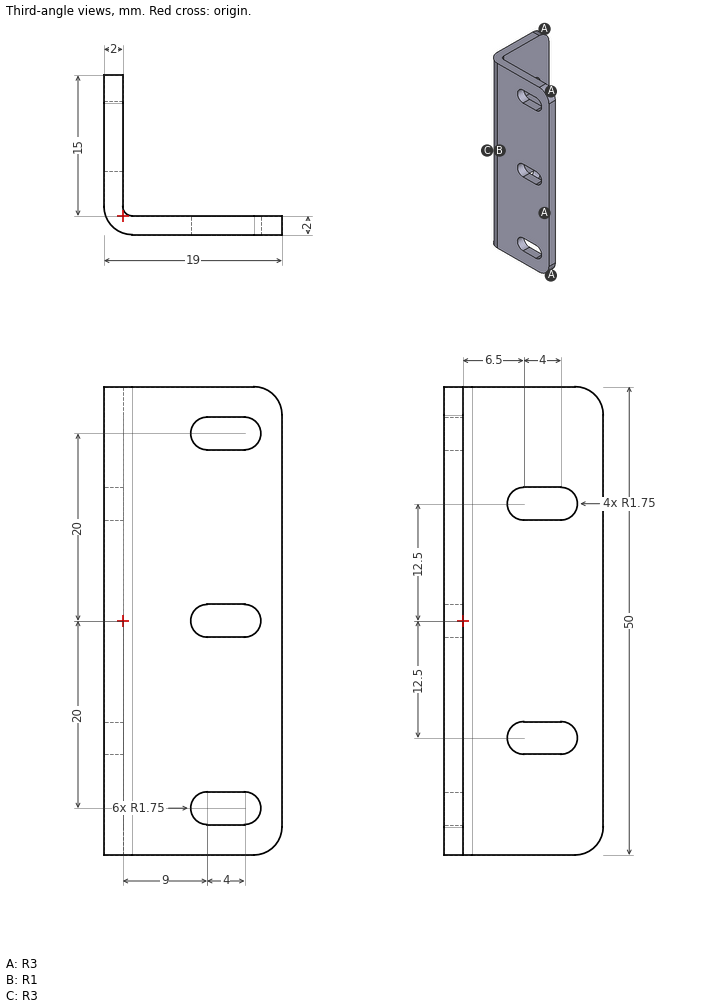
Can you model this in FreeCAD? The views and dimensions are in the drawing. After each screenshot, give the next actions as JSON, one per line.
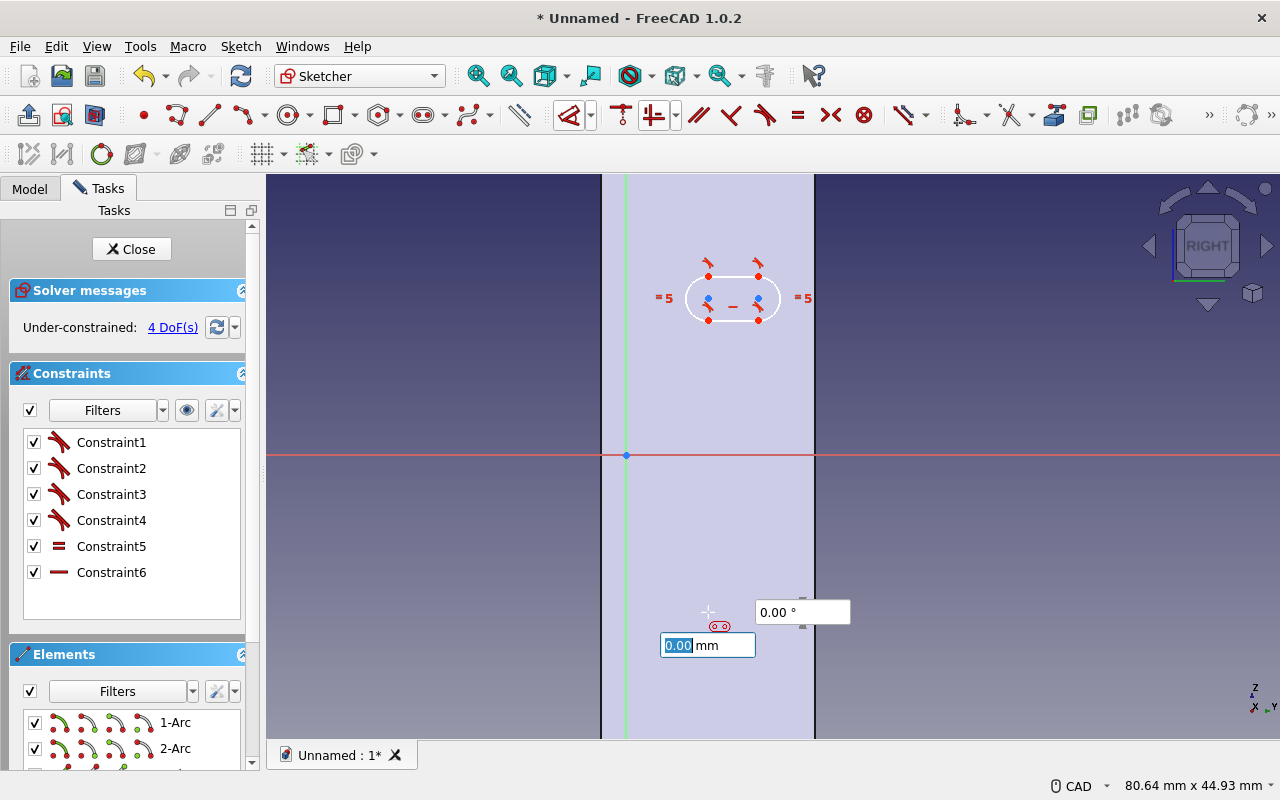
{"action": "left_click", "coordinate": [758, 612]}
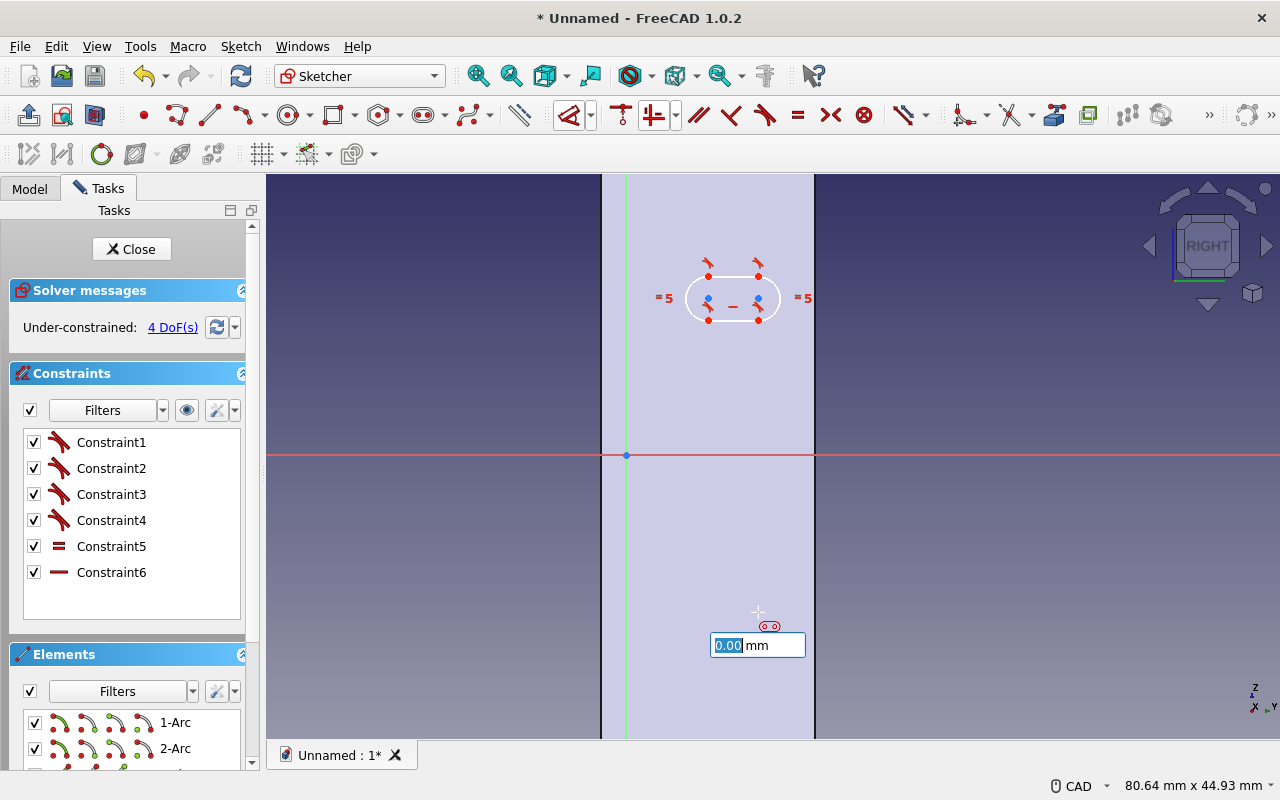
{"action": "left_click", "coordinate": [733, 590]}
{"action": "key", "text": "Escape"}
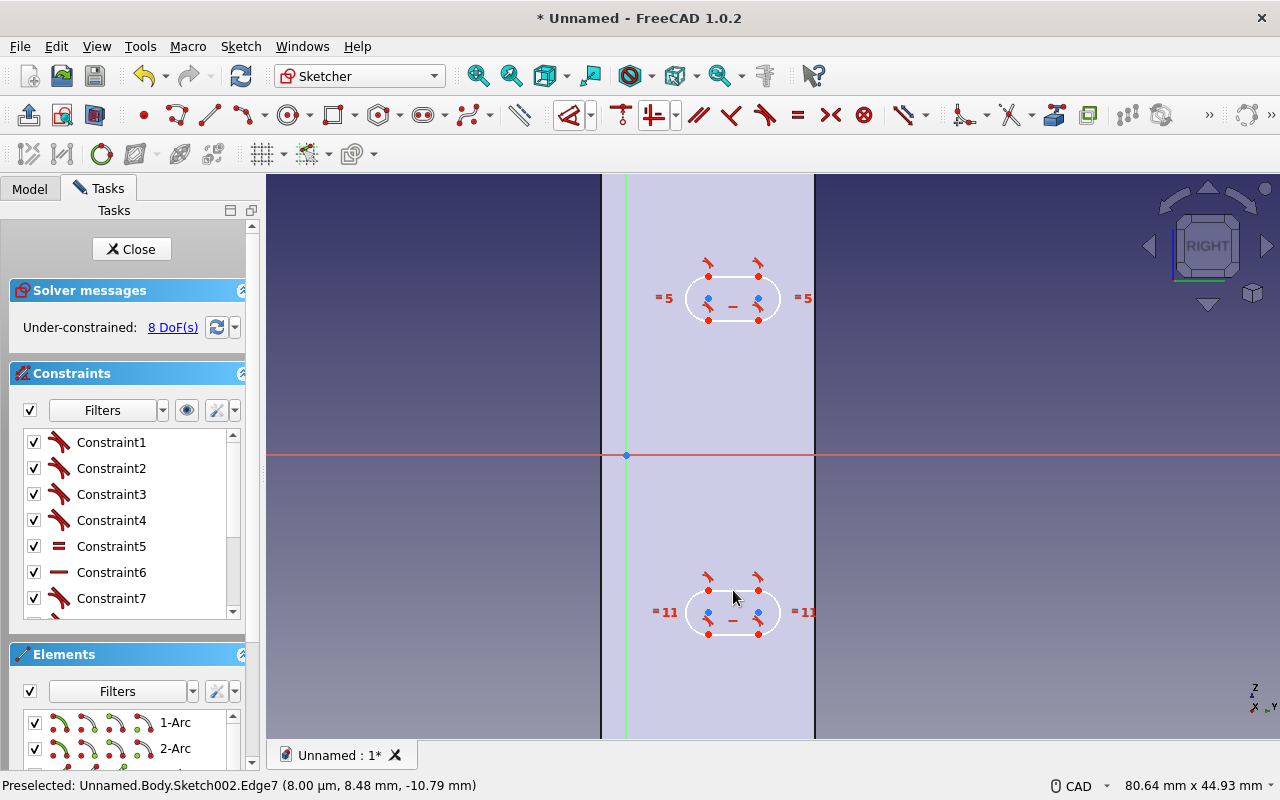
{"action": "left_click", "coordinate": [690, 286]}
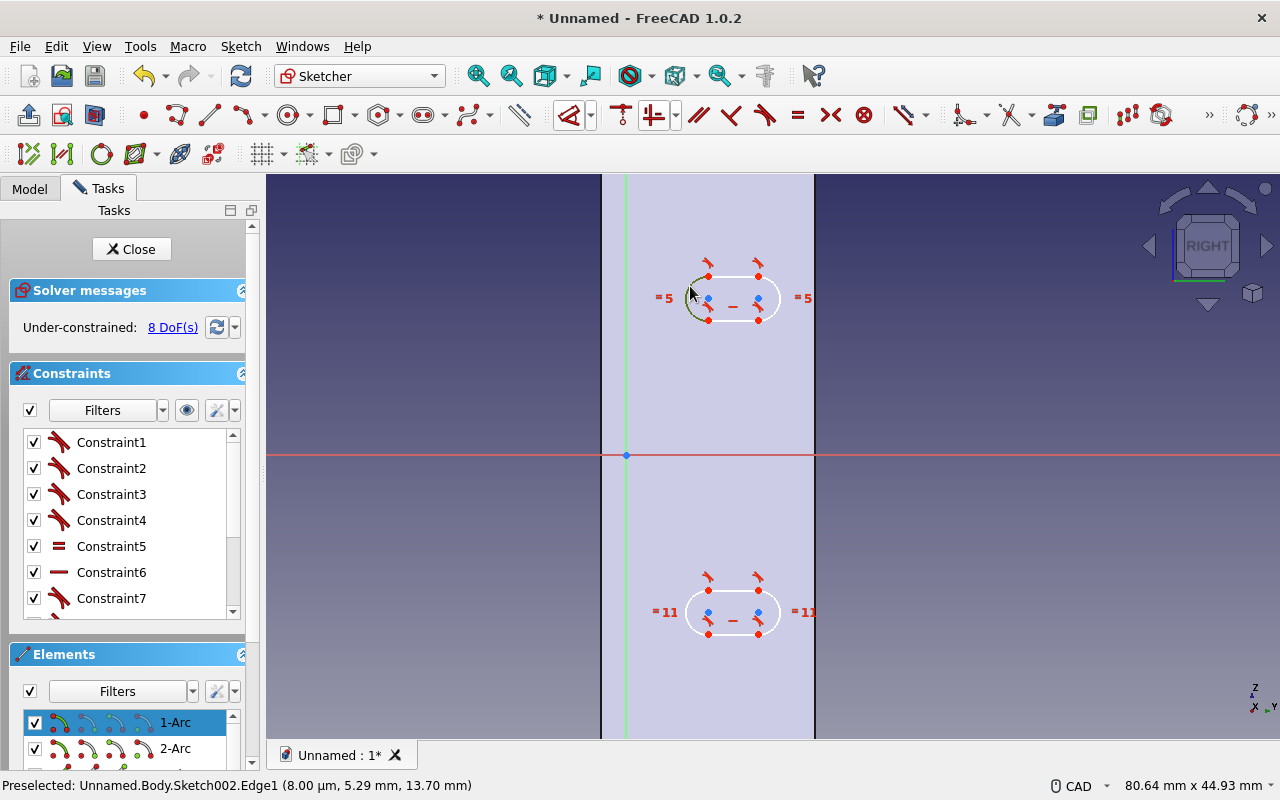
{"action": "left_click", "coordinate": [690, 600]}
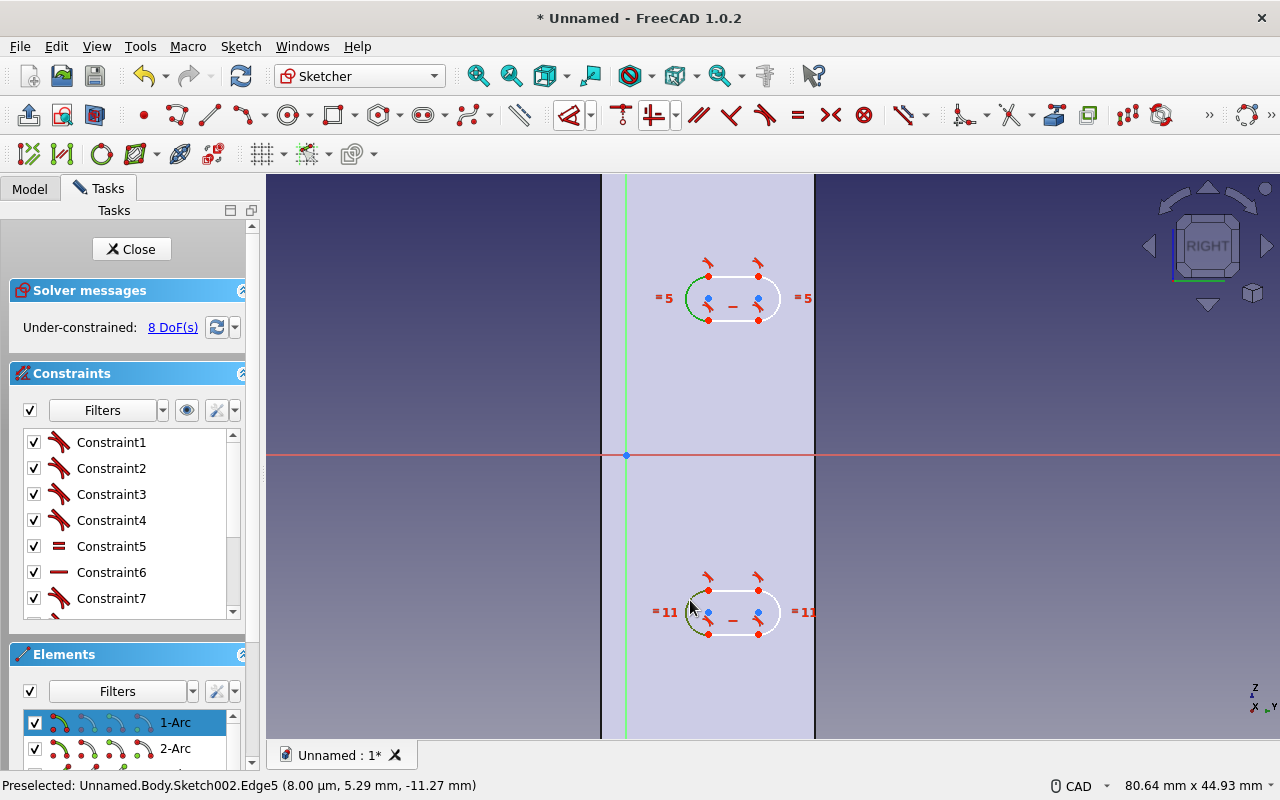
{"action": "left_click", "coordinate": [798, 116]}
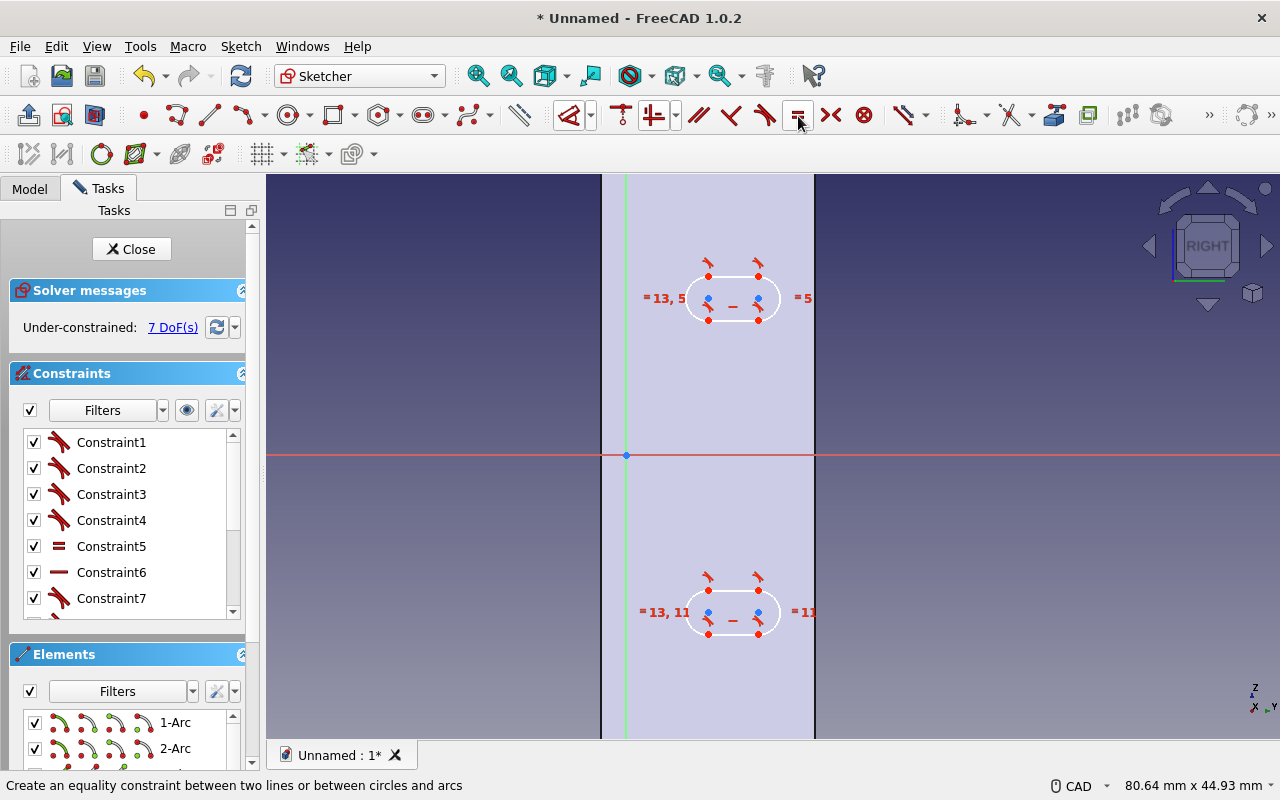
{"action": "scroll", "coordinate": [690, 286], "scroll_direction": "up", "scroll_amount": 3}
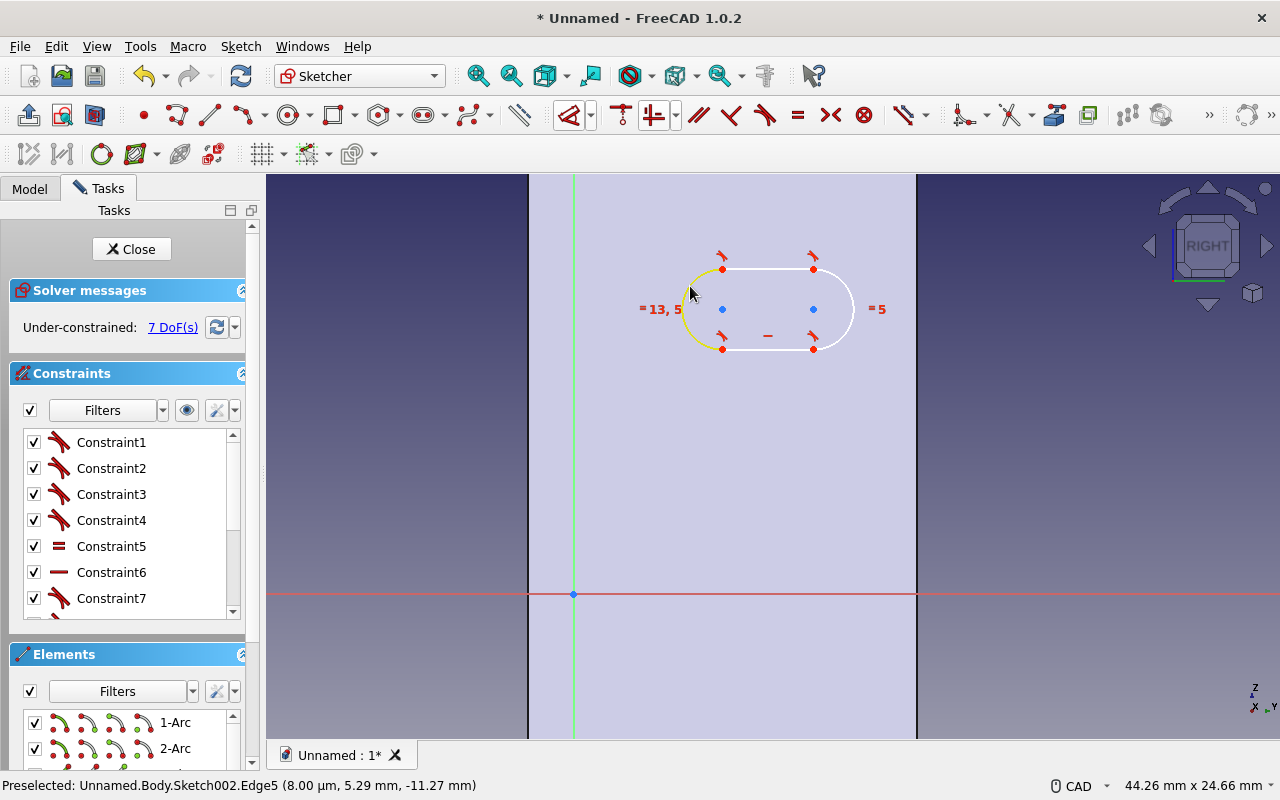
{"action": "left_click", "coordinate": [690, 286]}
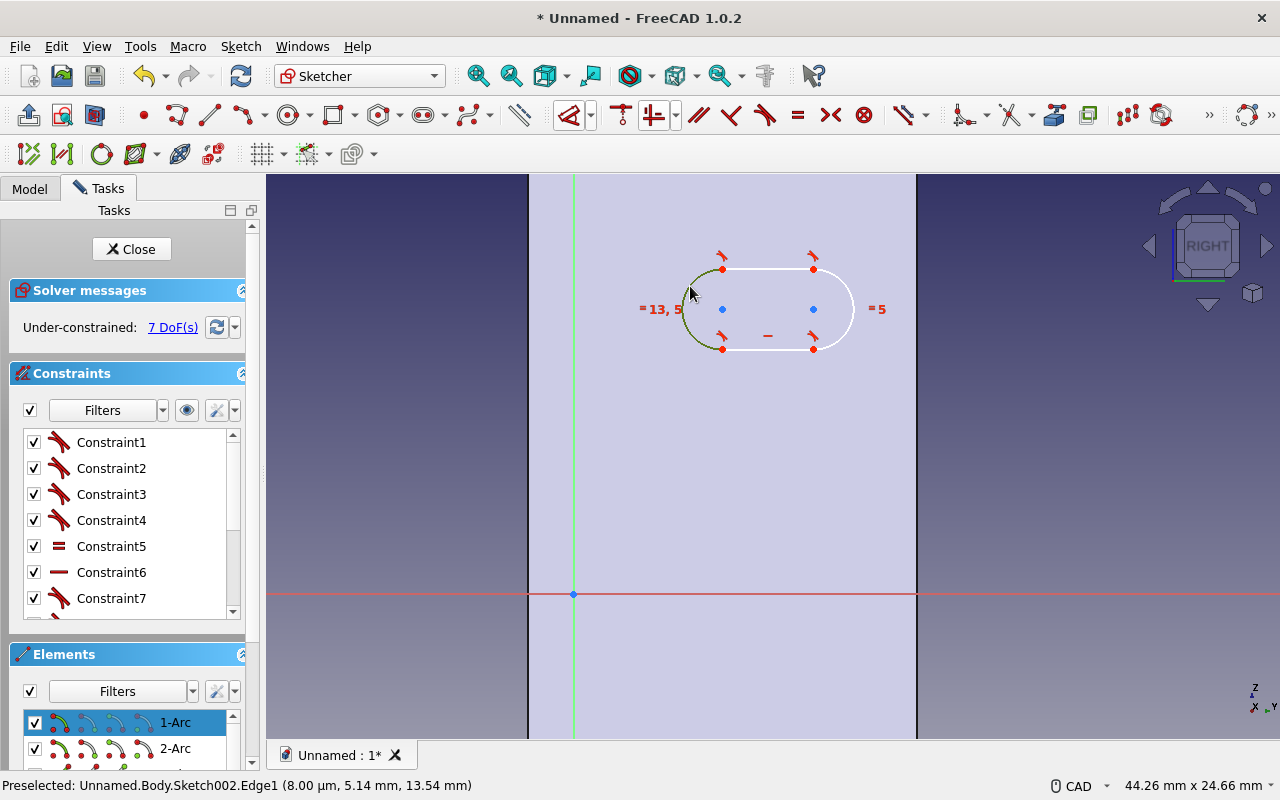
{"action": "left_click", "coordinate": [590, 116]}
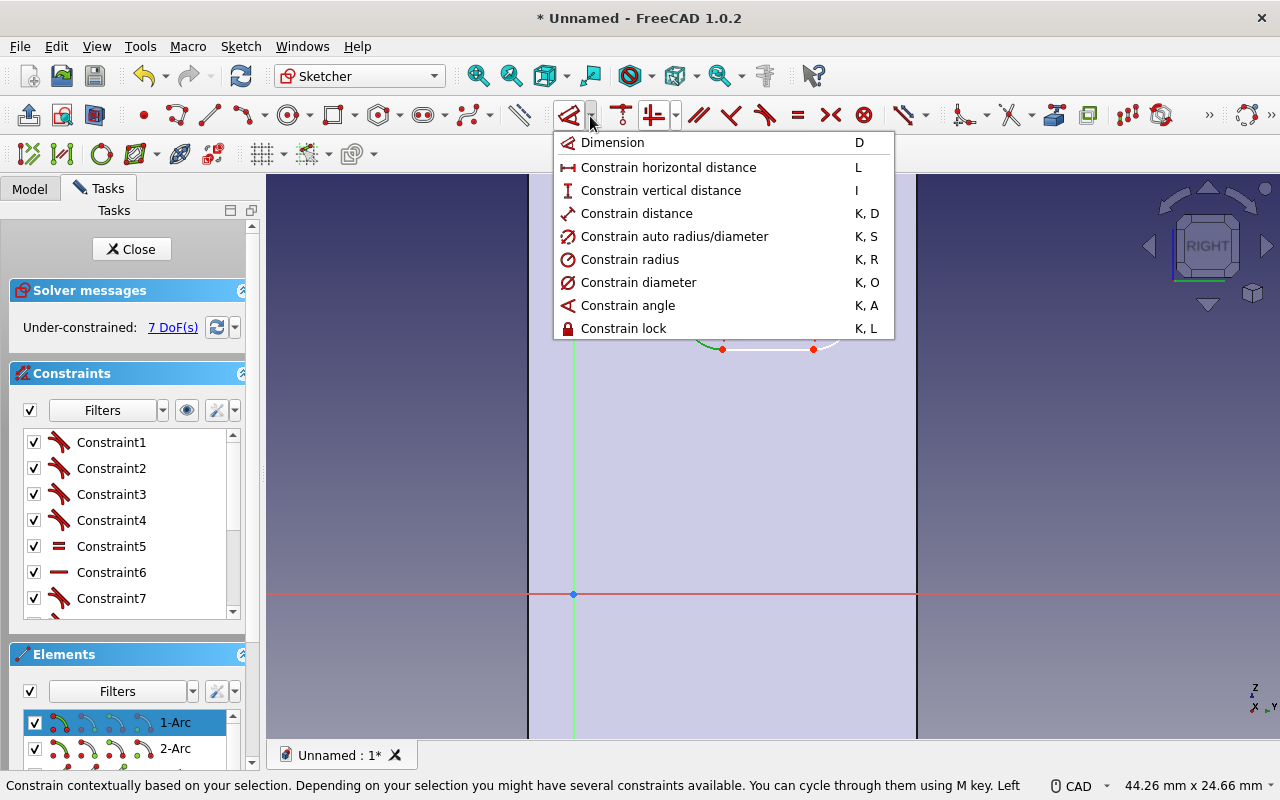
{"action": "left_click", "coordinate": [724, 260]}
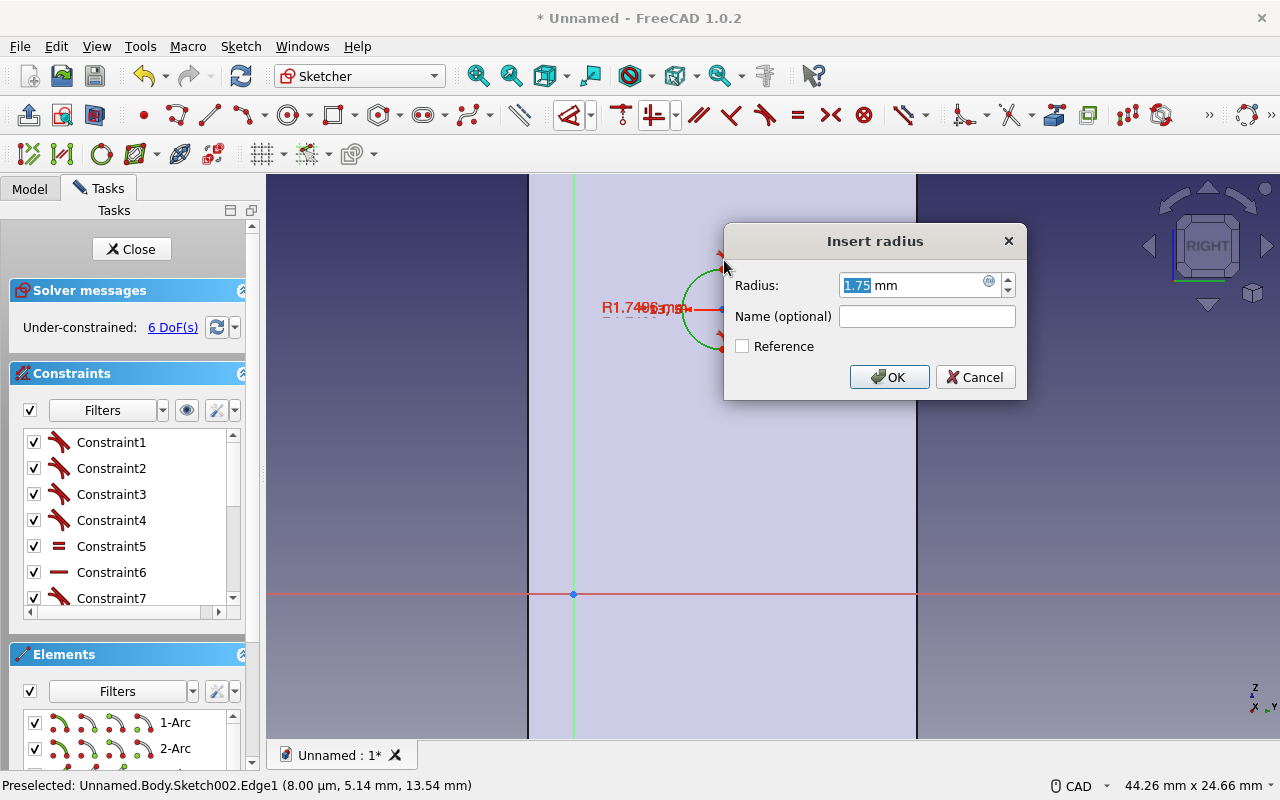
{"action": "type", "text": "1.75"}
{"action": "key", "text": "Return"}